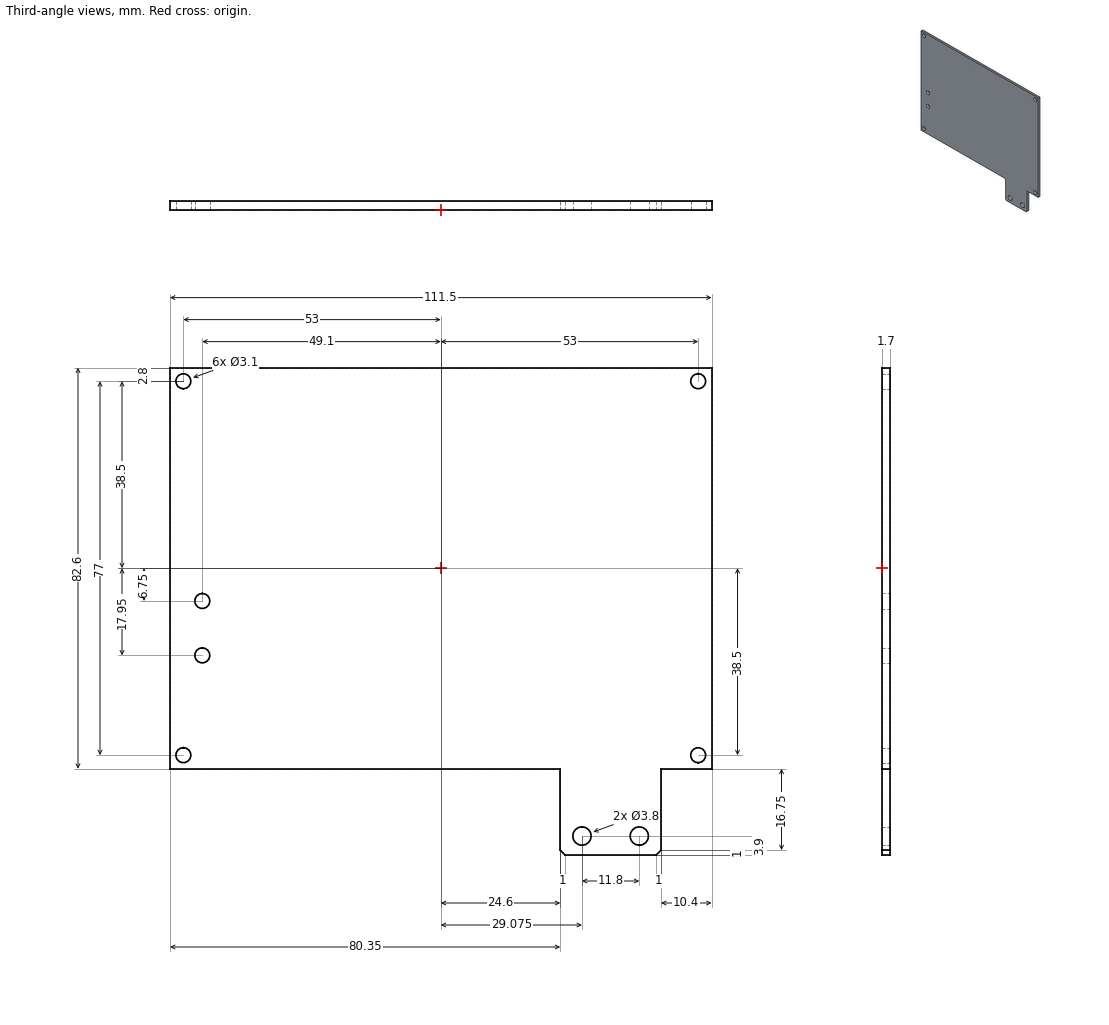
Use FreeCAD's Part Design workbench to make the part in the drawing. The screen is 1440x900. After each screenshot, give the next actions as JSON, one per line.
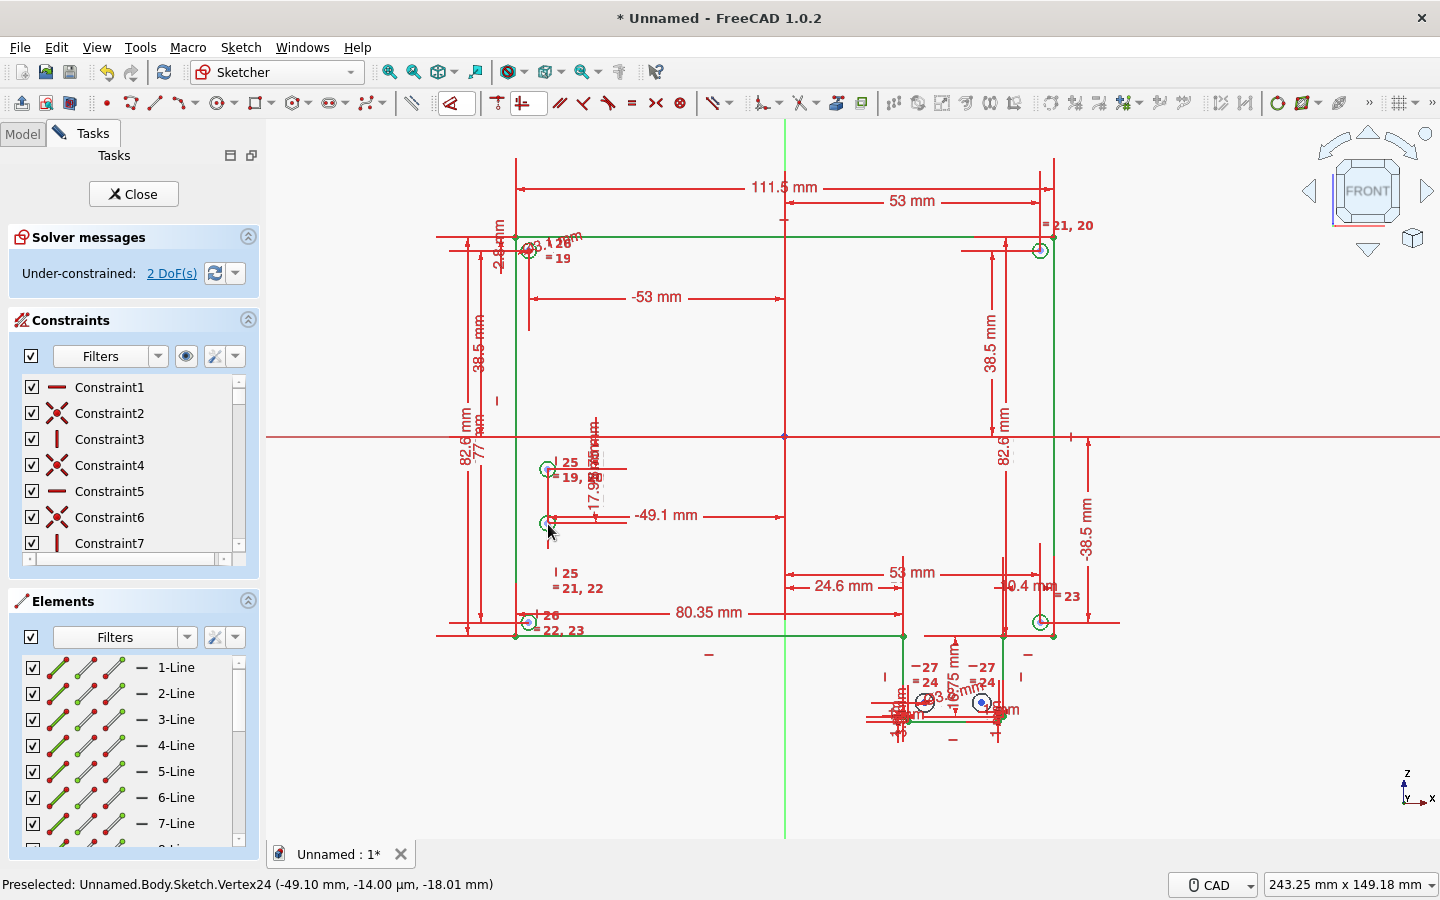
{"action": "left_click", "coordinate": [925, 703]}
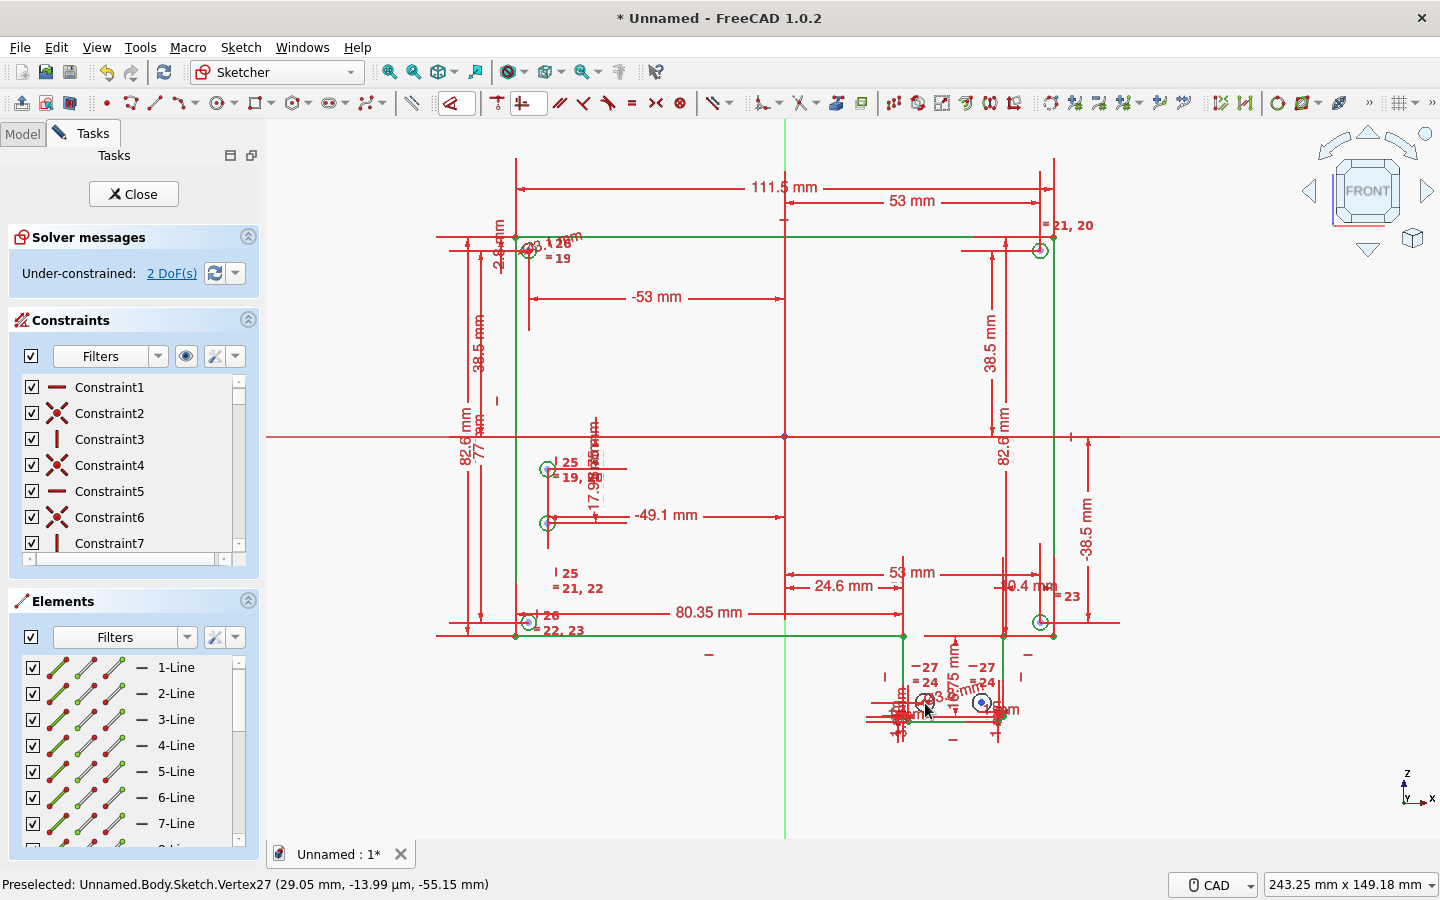
{"action": "left_click", "coordinate": [982, 703]}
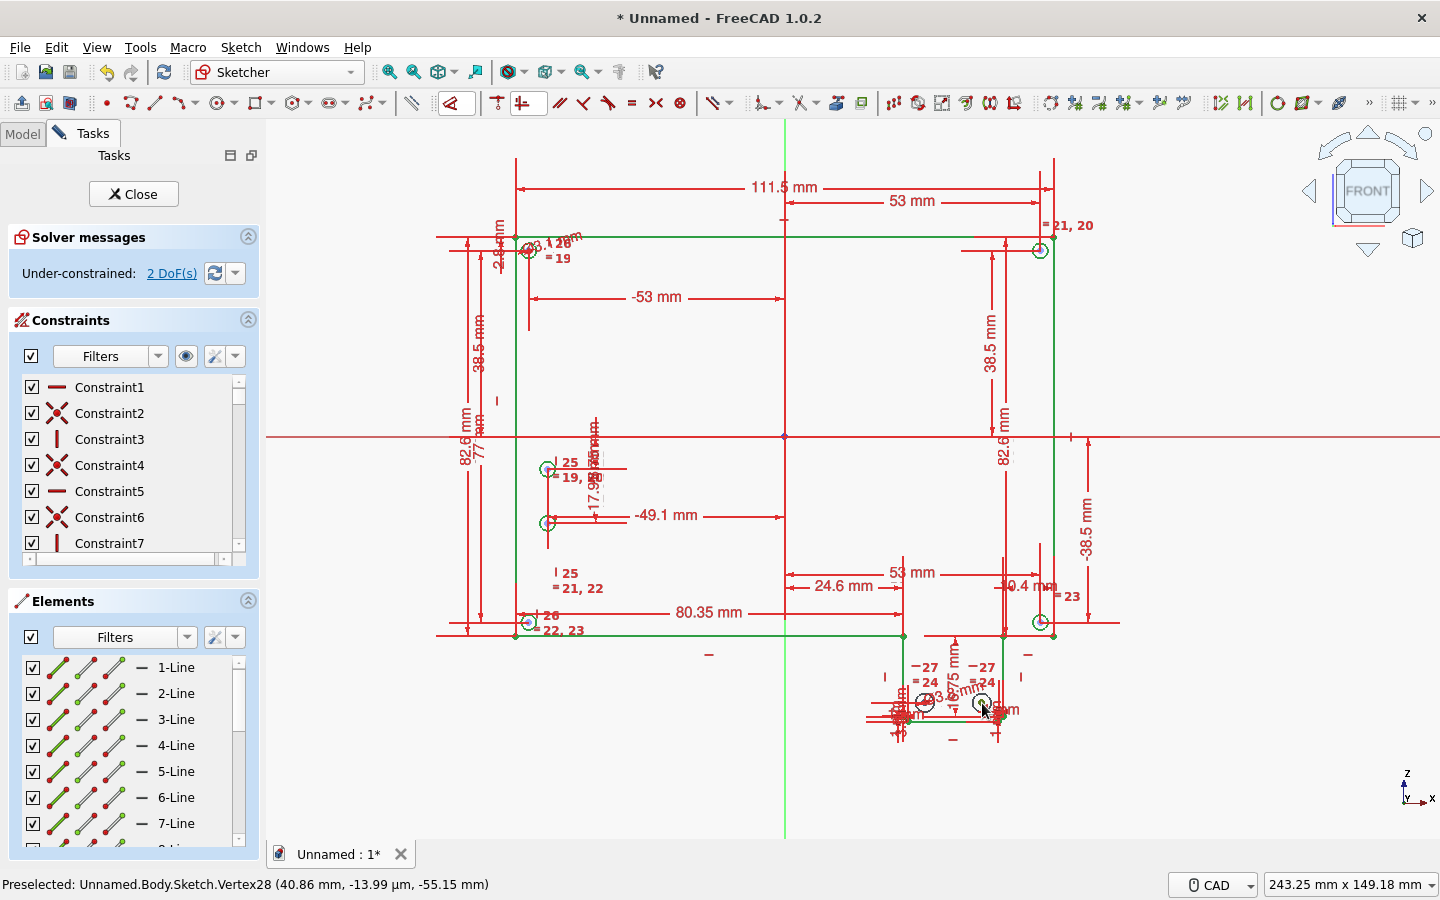
{"action": "key", "text": "l"}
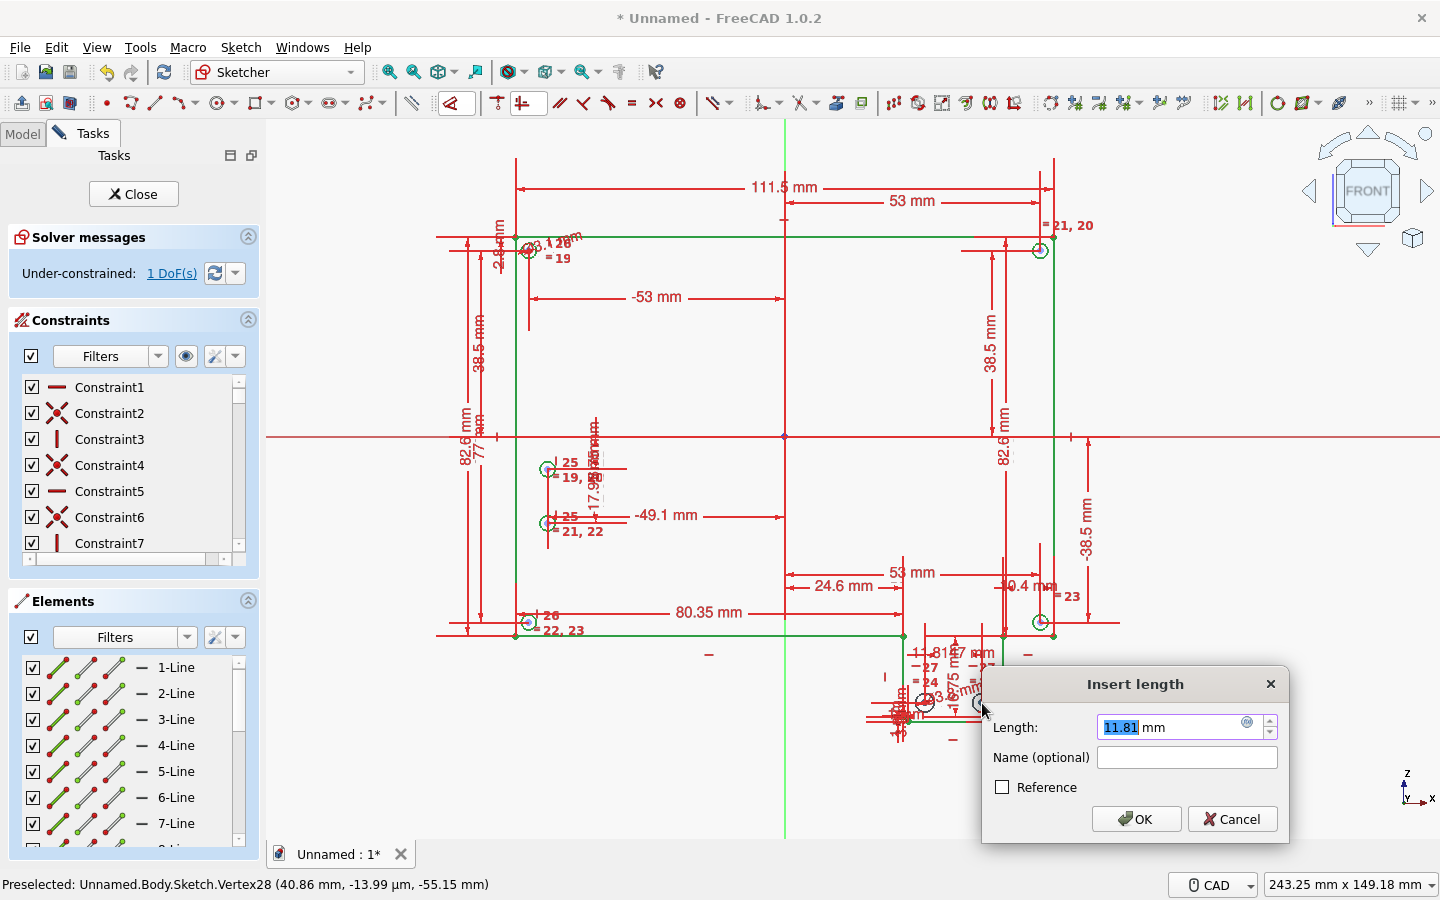
{"action": "type", "text": "11.8"}
{"action": "key", "text": "Return"}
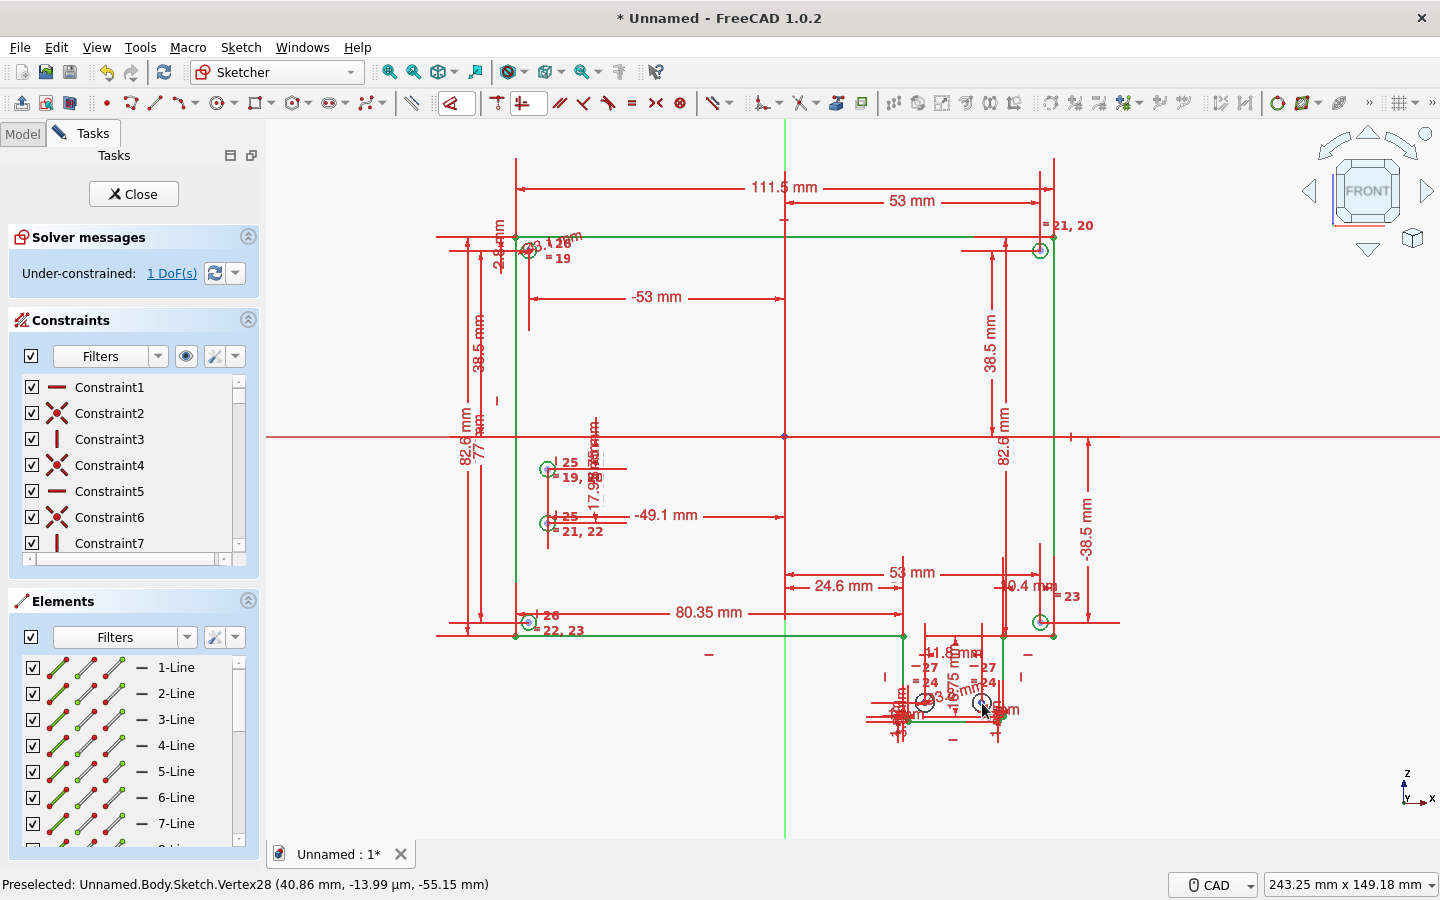
{"action": "left_click", "coordinate": [925, 703]}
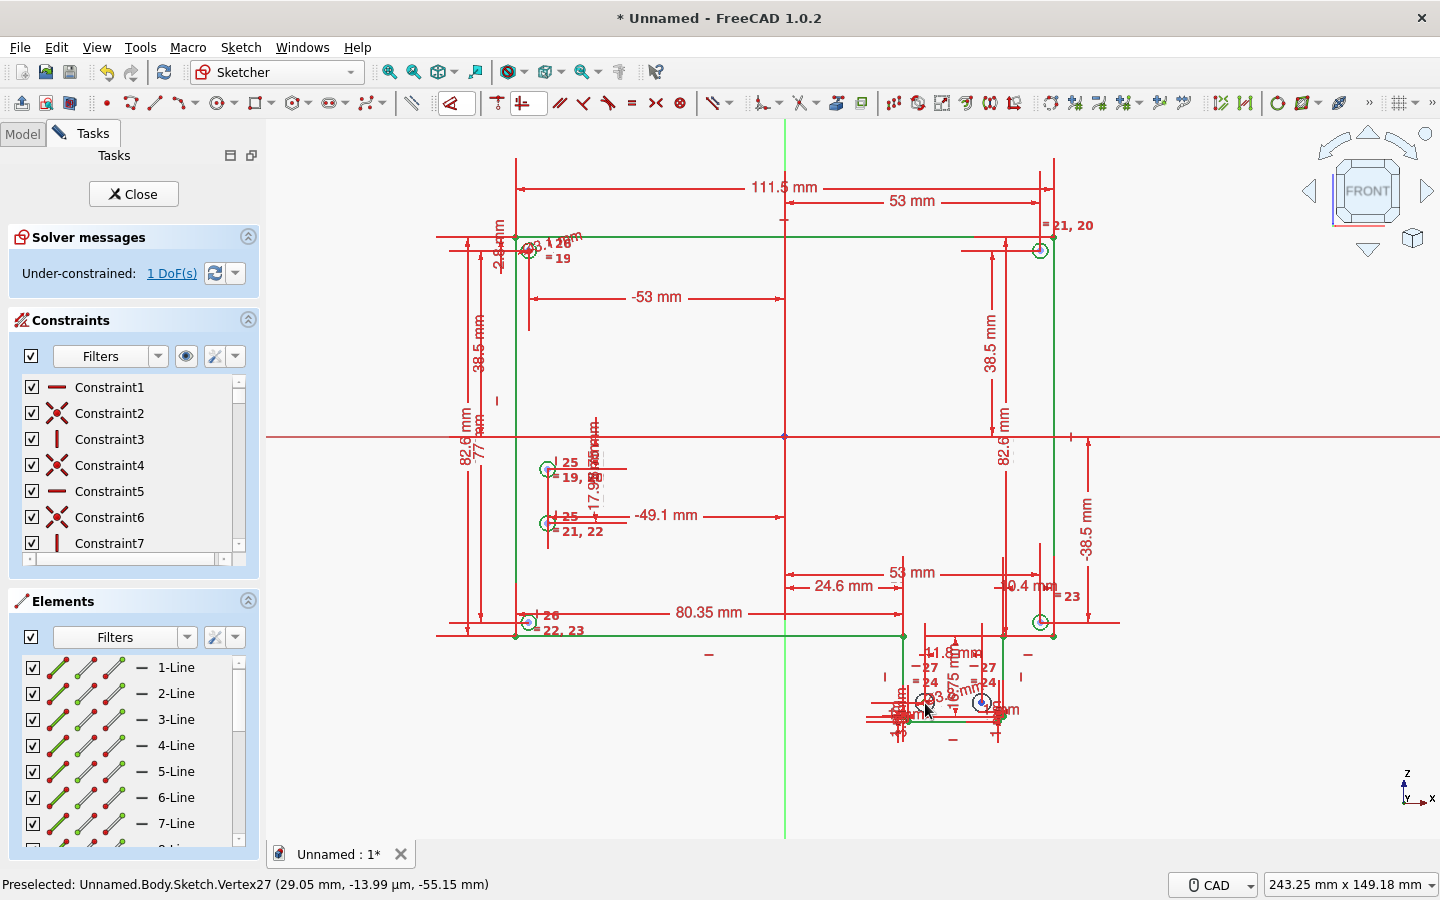
{"action": "key", "text": "l"}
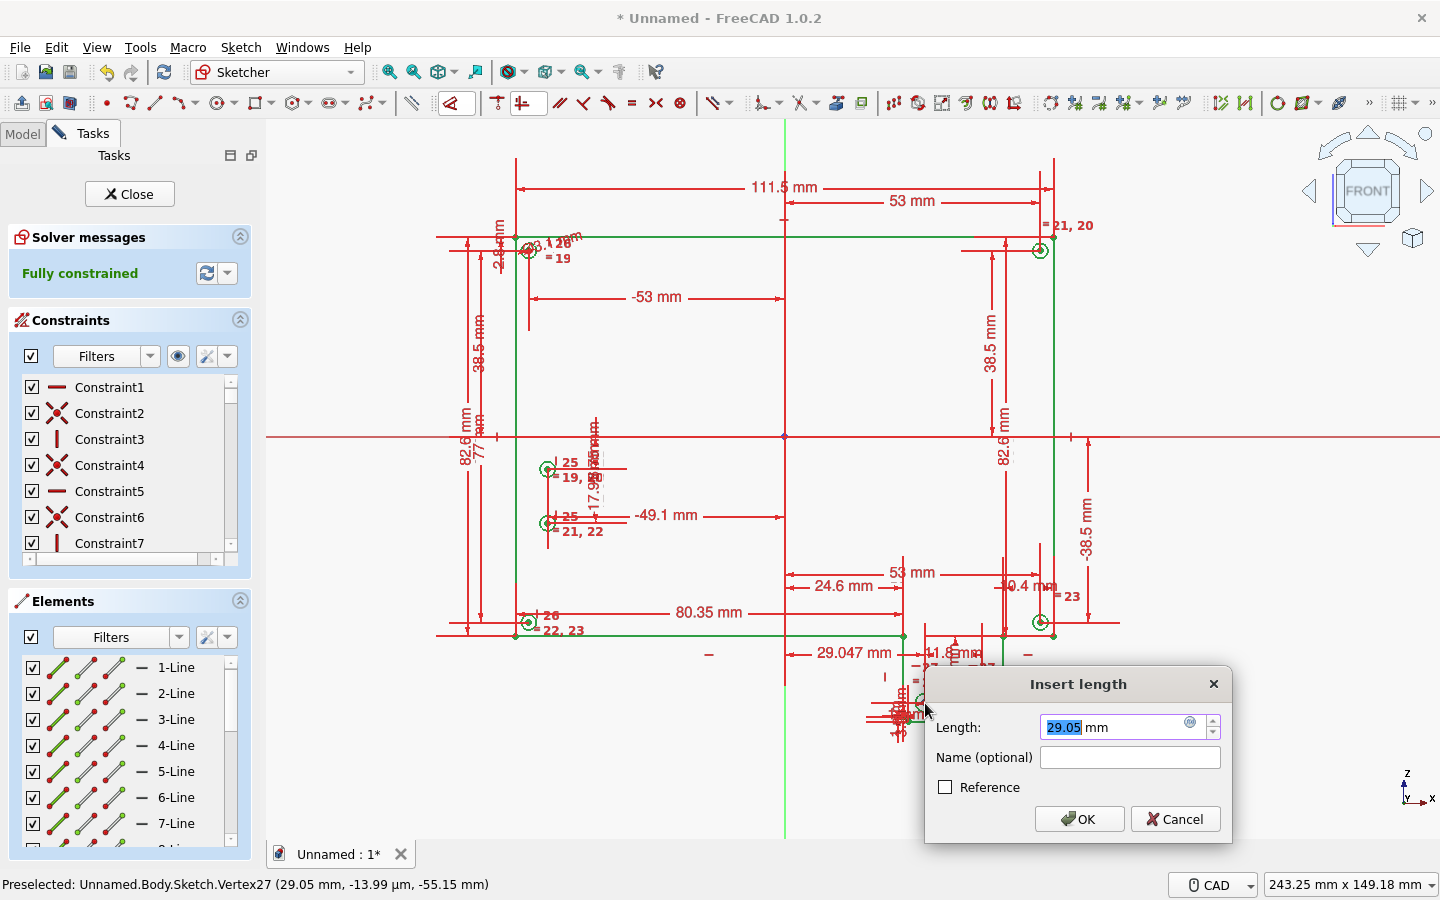
{"action": "type", "text": "29.075"}
{"action": "key", "text": "Return"}